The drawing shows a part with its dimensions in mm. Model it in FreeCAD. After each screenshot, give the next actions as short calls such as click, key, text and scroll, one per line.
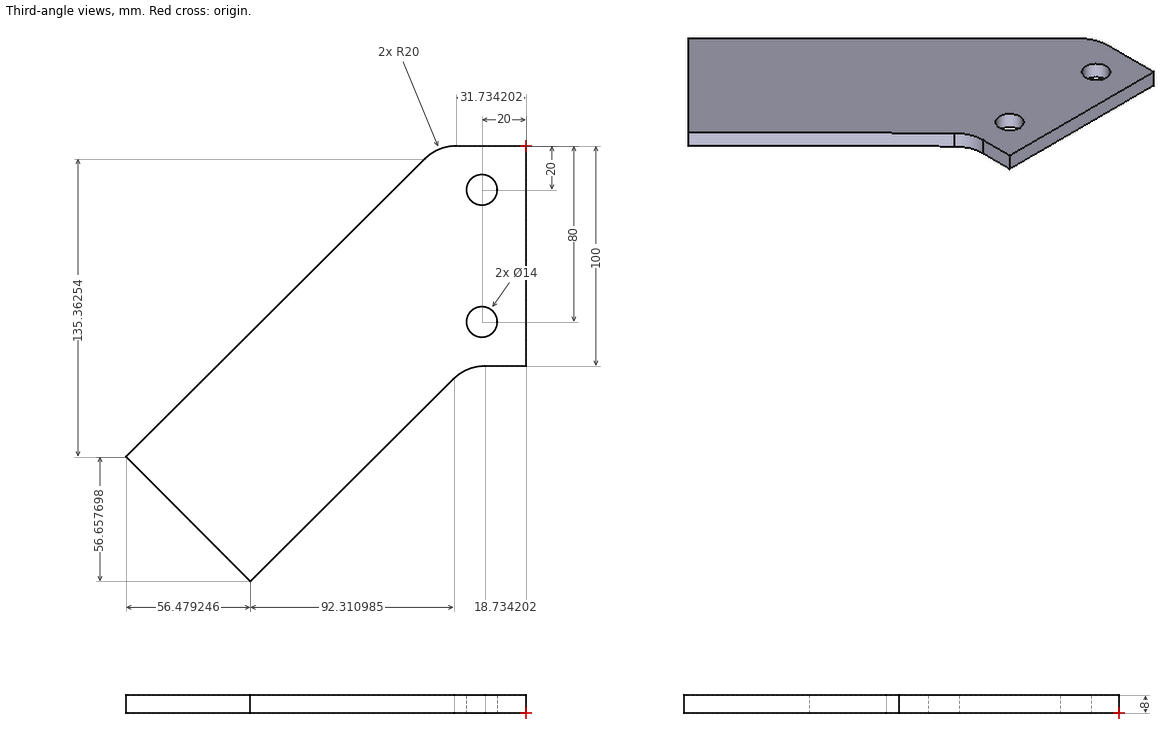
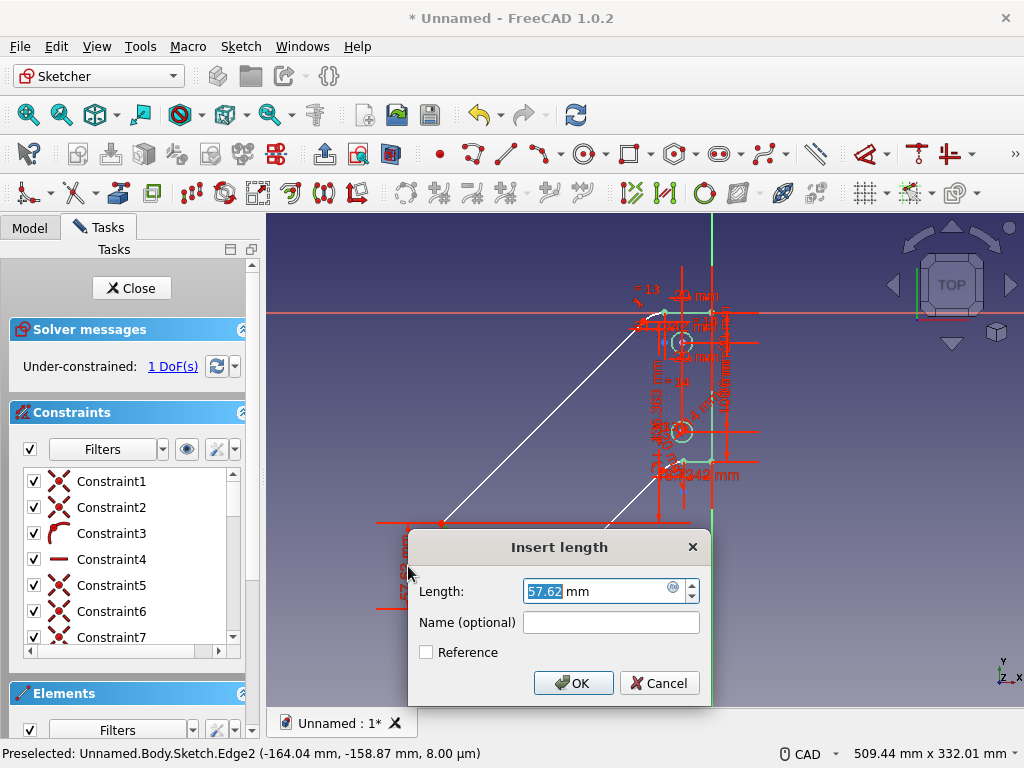
text(56.657698)
key(Return)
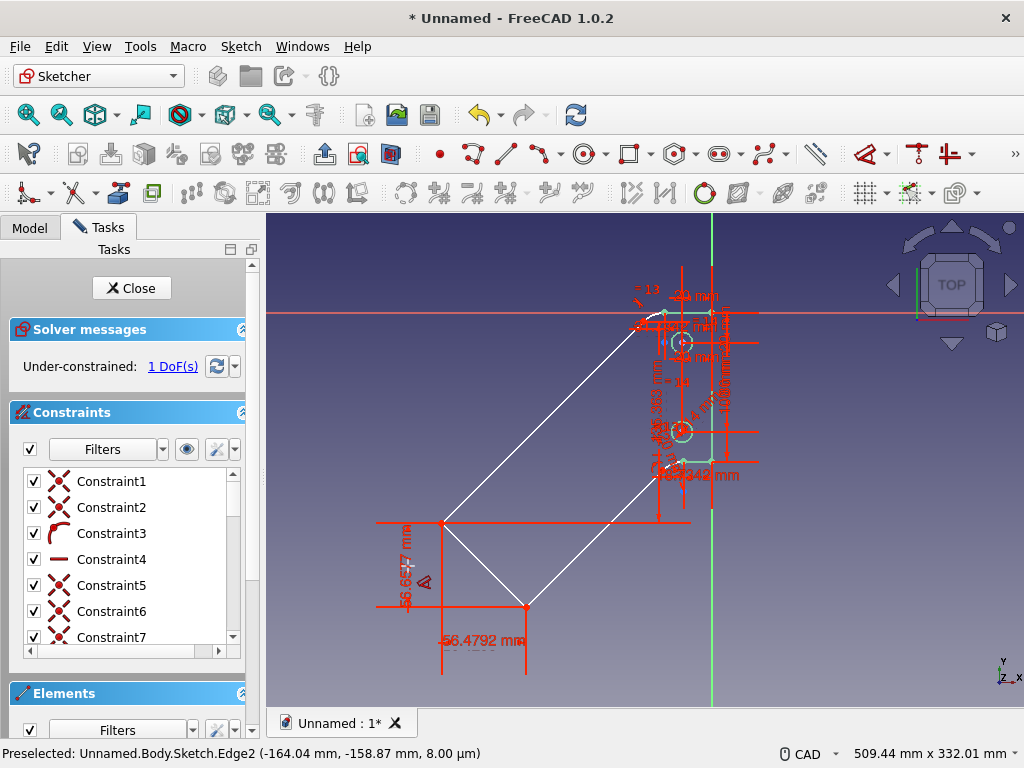
click(567, 566)
click(594, 641)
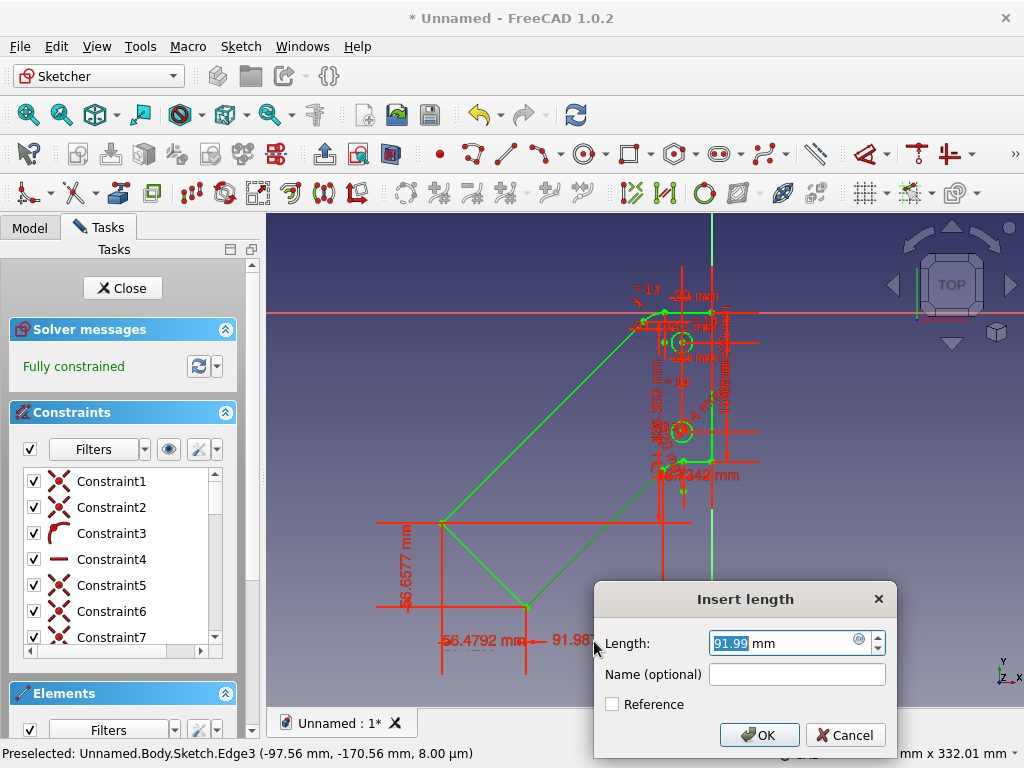
text(92.310985)
key(Return)
key(Escape)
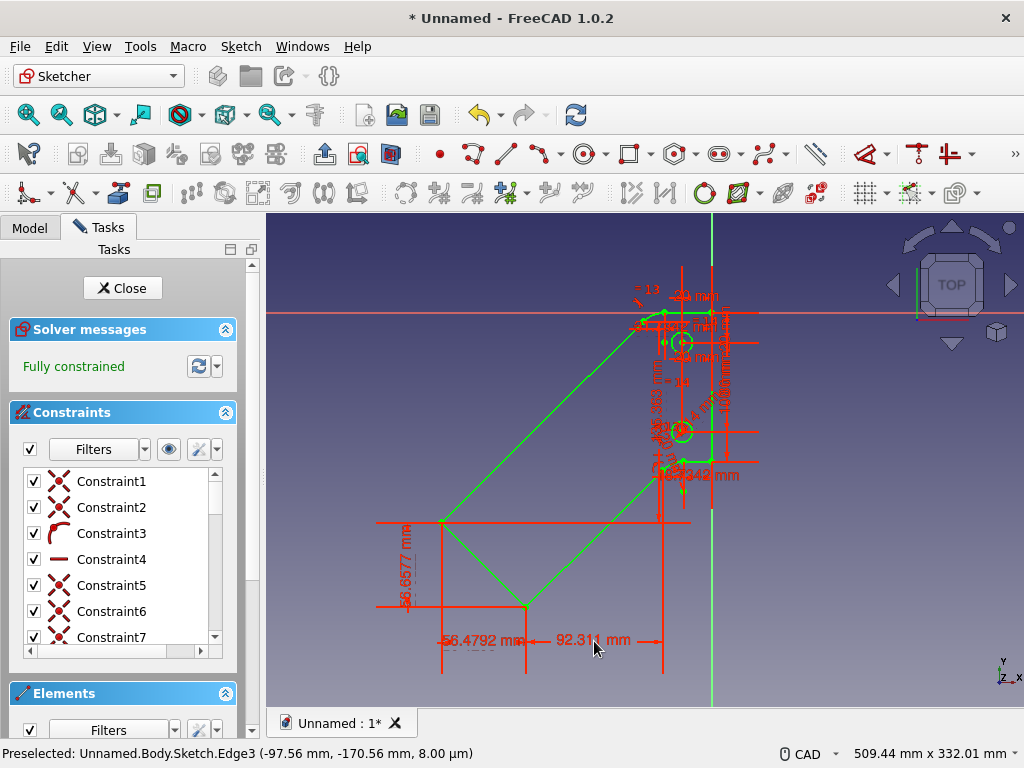
click(123, 288)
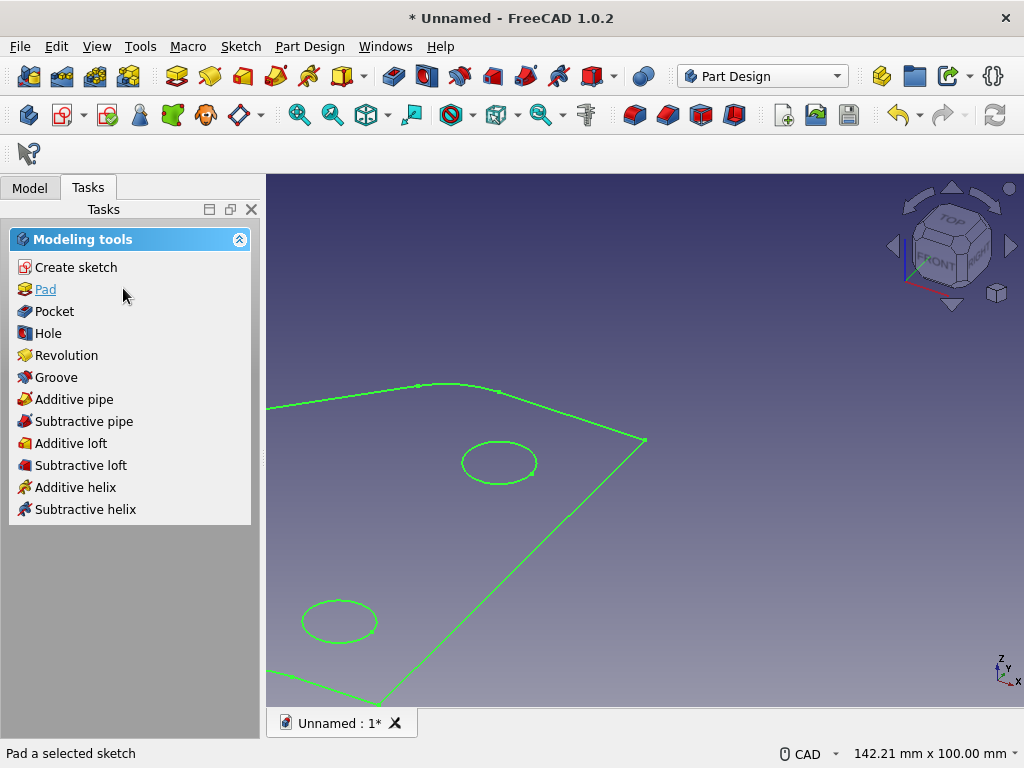
click(177, 76)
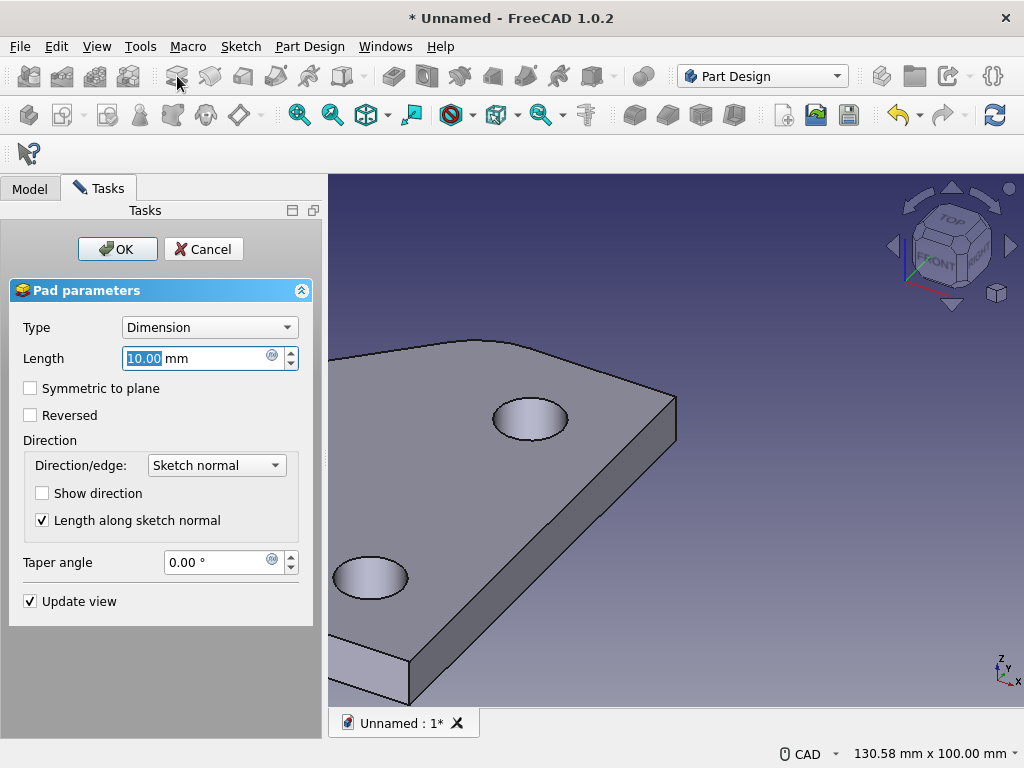
text(8)
key(Tab)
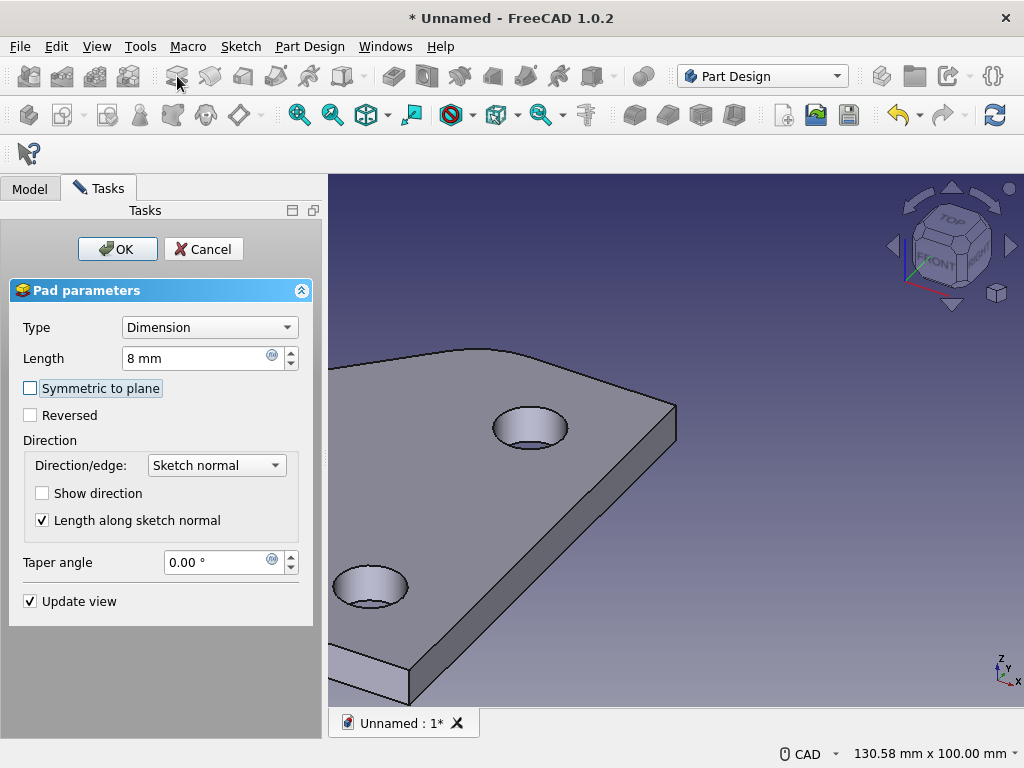
click(118, 249)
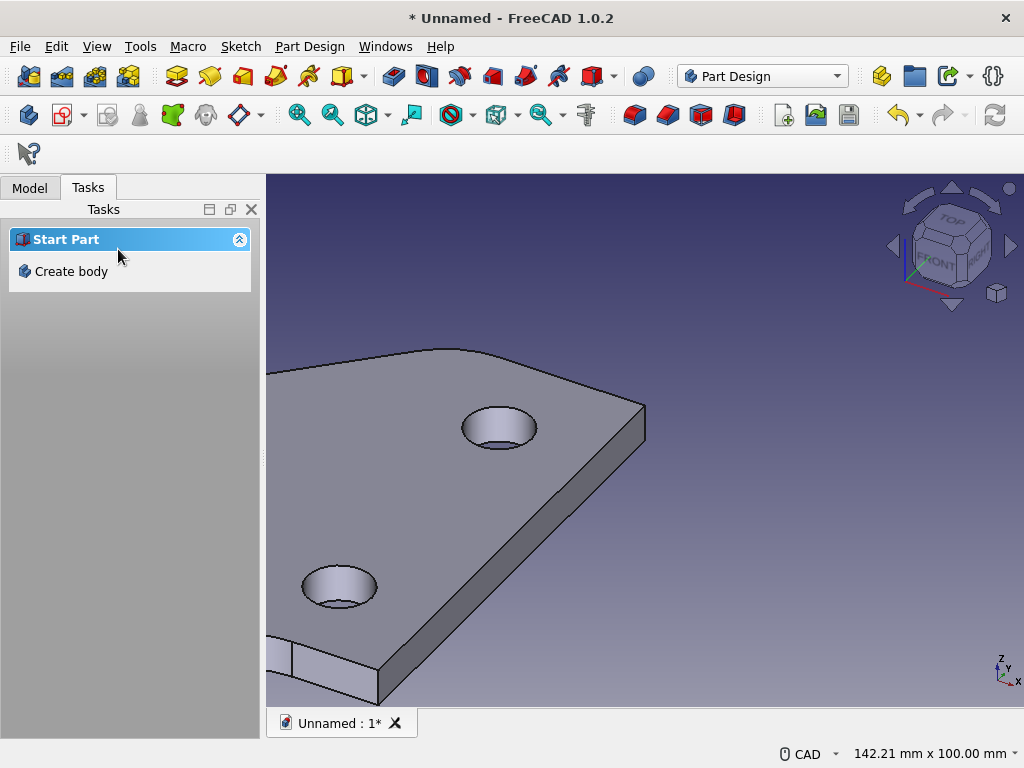
key(0)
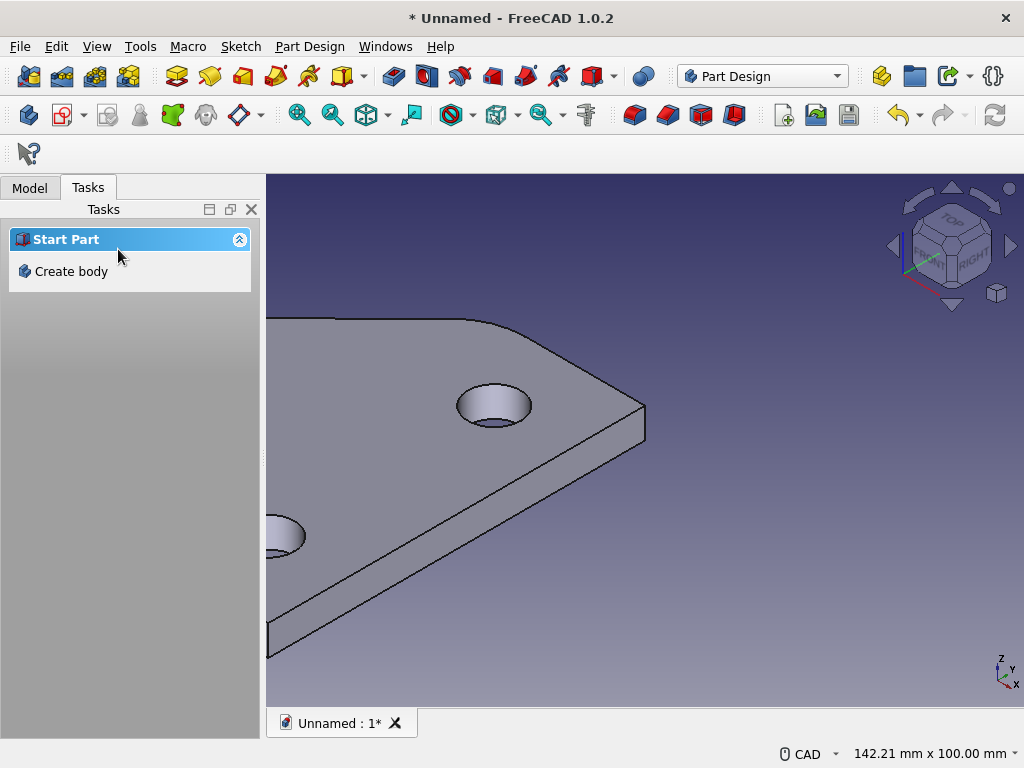
click(300, 116)